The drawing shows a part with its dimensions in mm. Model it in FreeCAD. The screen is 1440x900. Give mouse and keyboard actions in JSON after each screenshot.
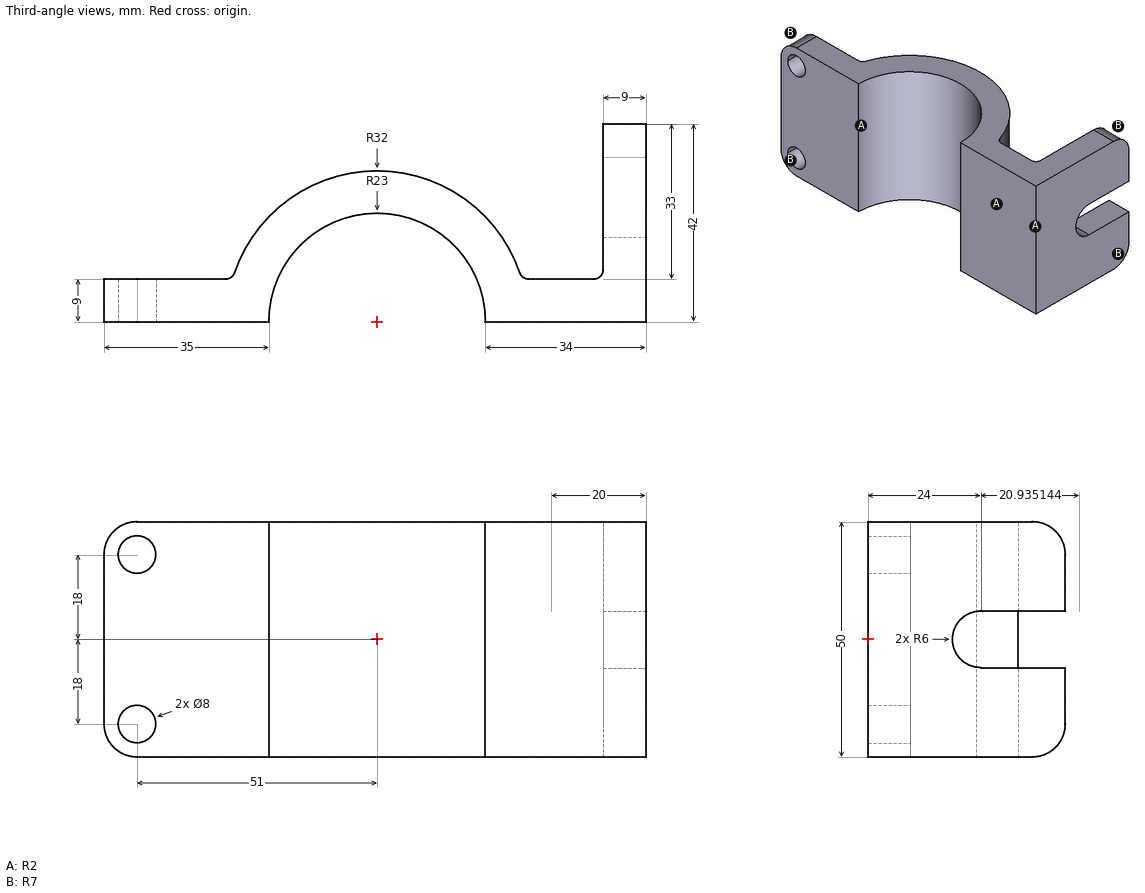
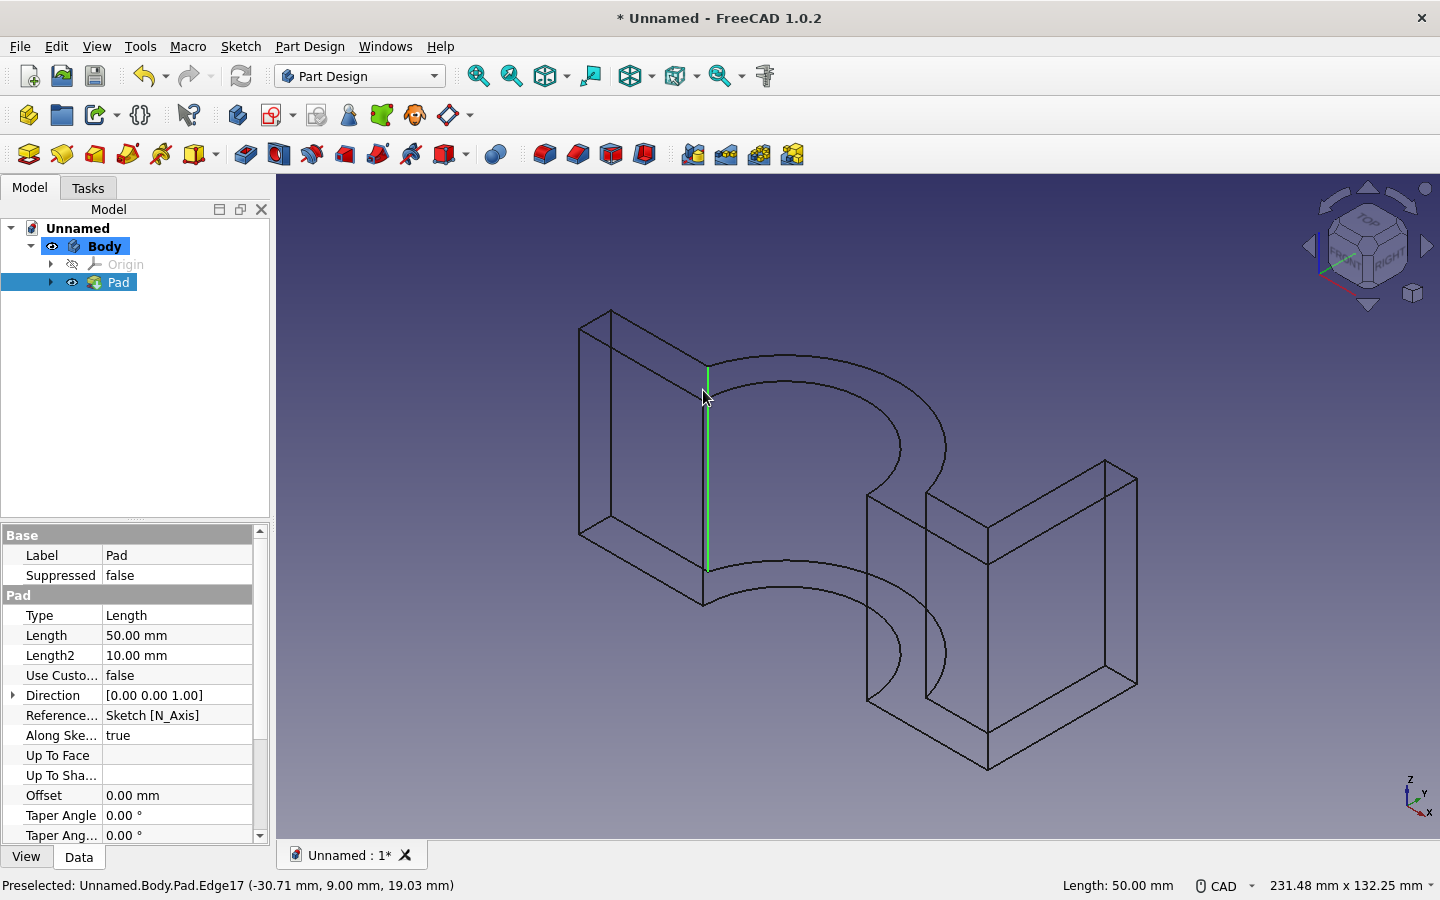
{"action": "left_click", "coordinate": [926, 594], "text": "ctrl"}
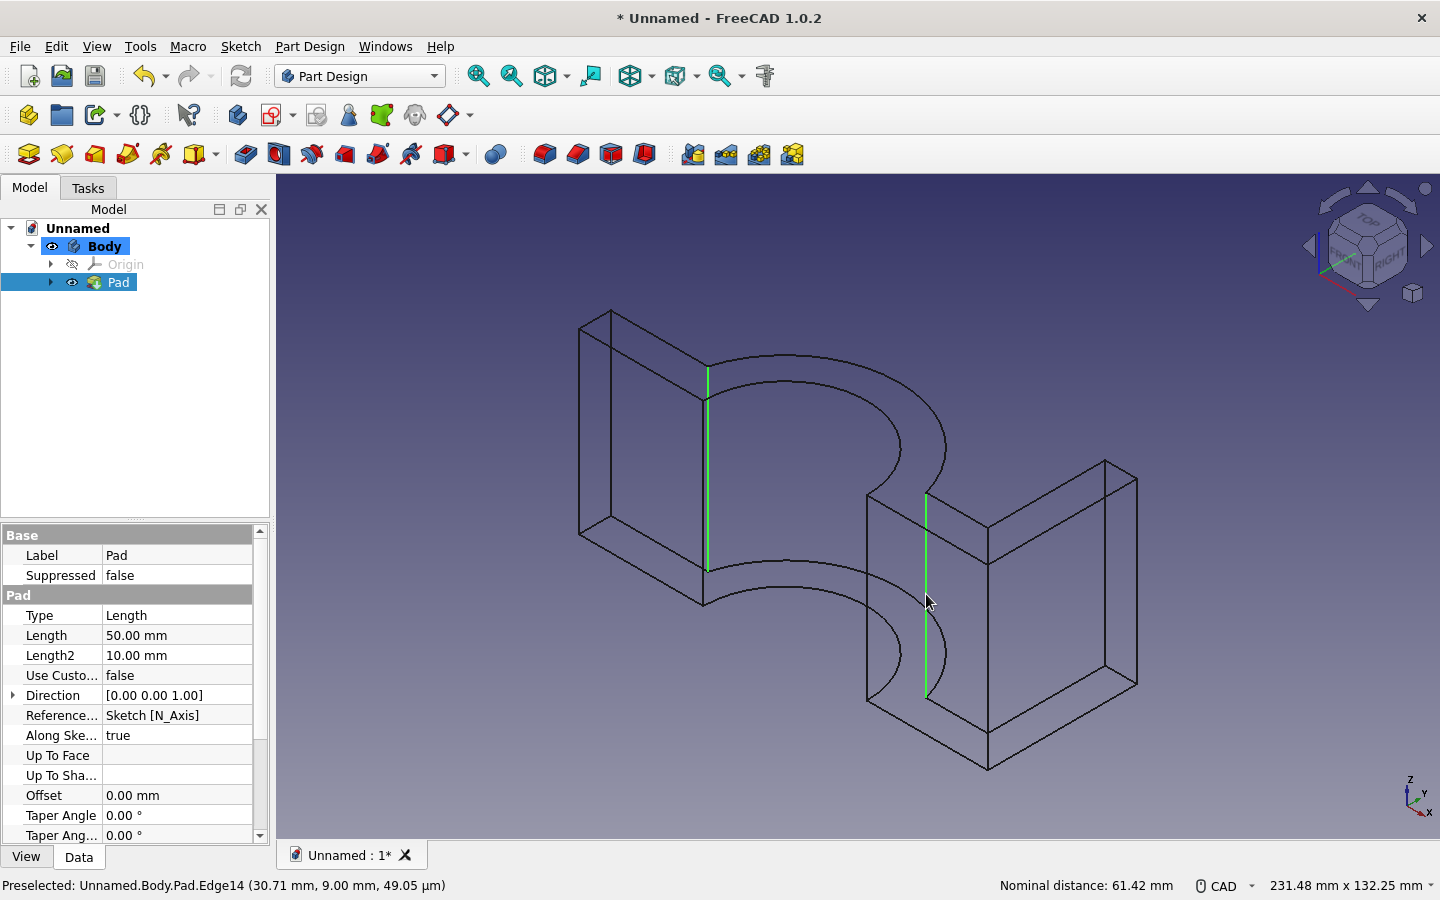
{"action": "left_click", "coordinate": [988, 552], "text": "ctrl"}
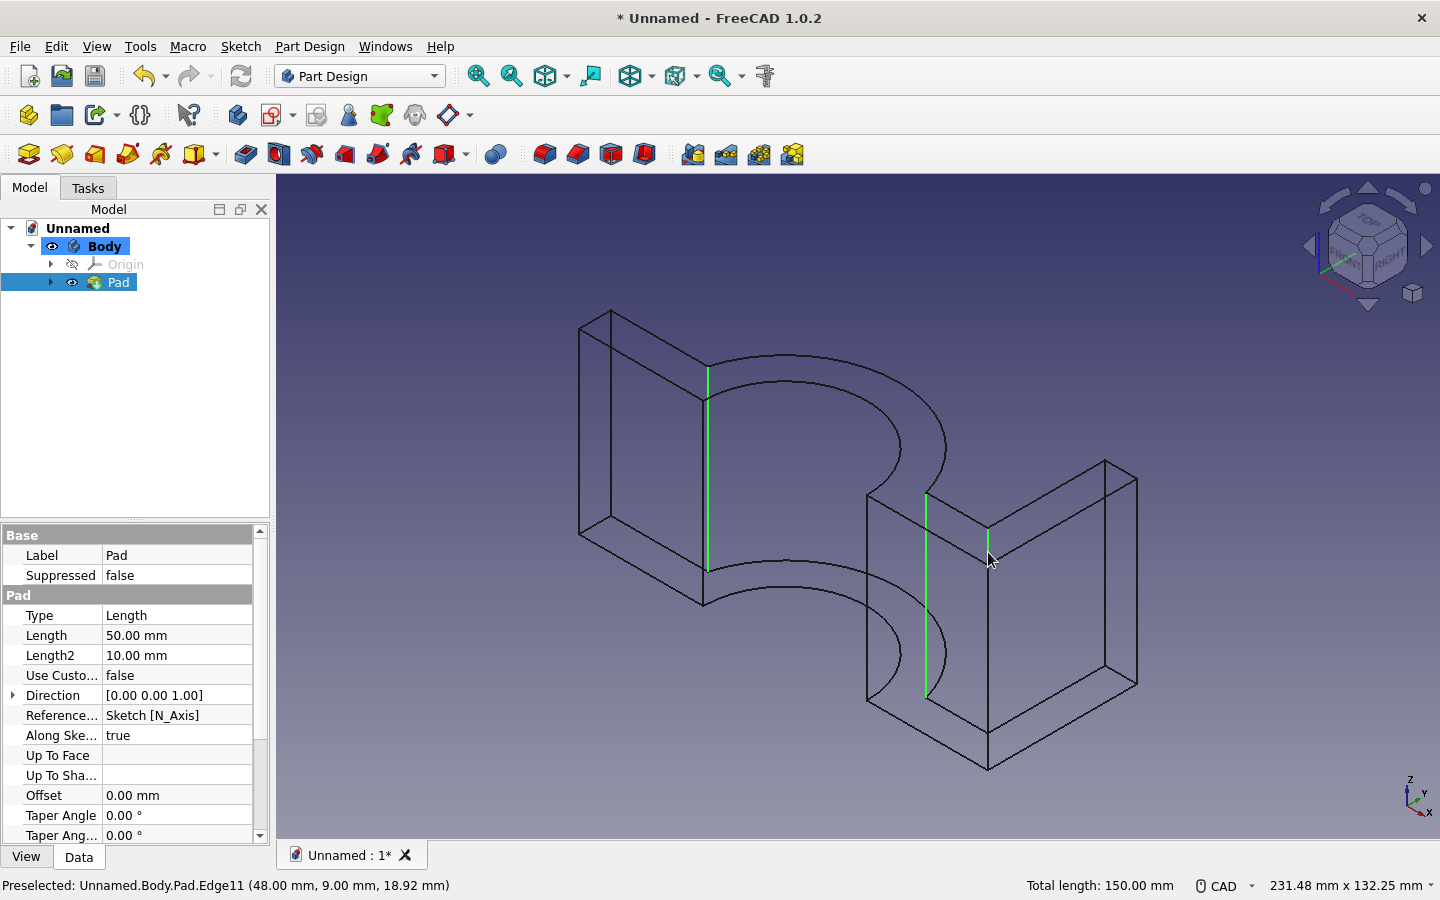
{"action": "key", "text": "v 1"}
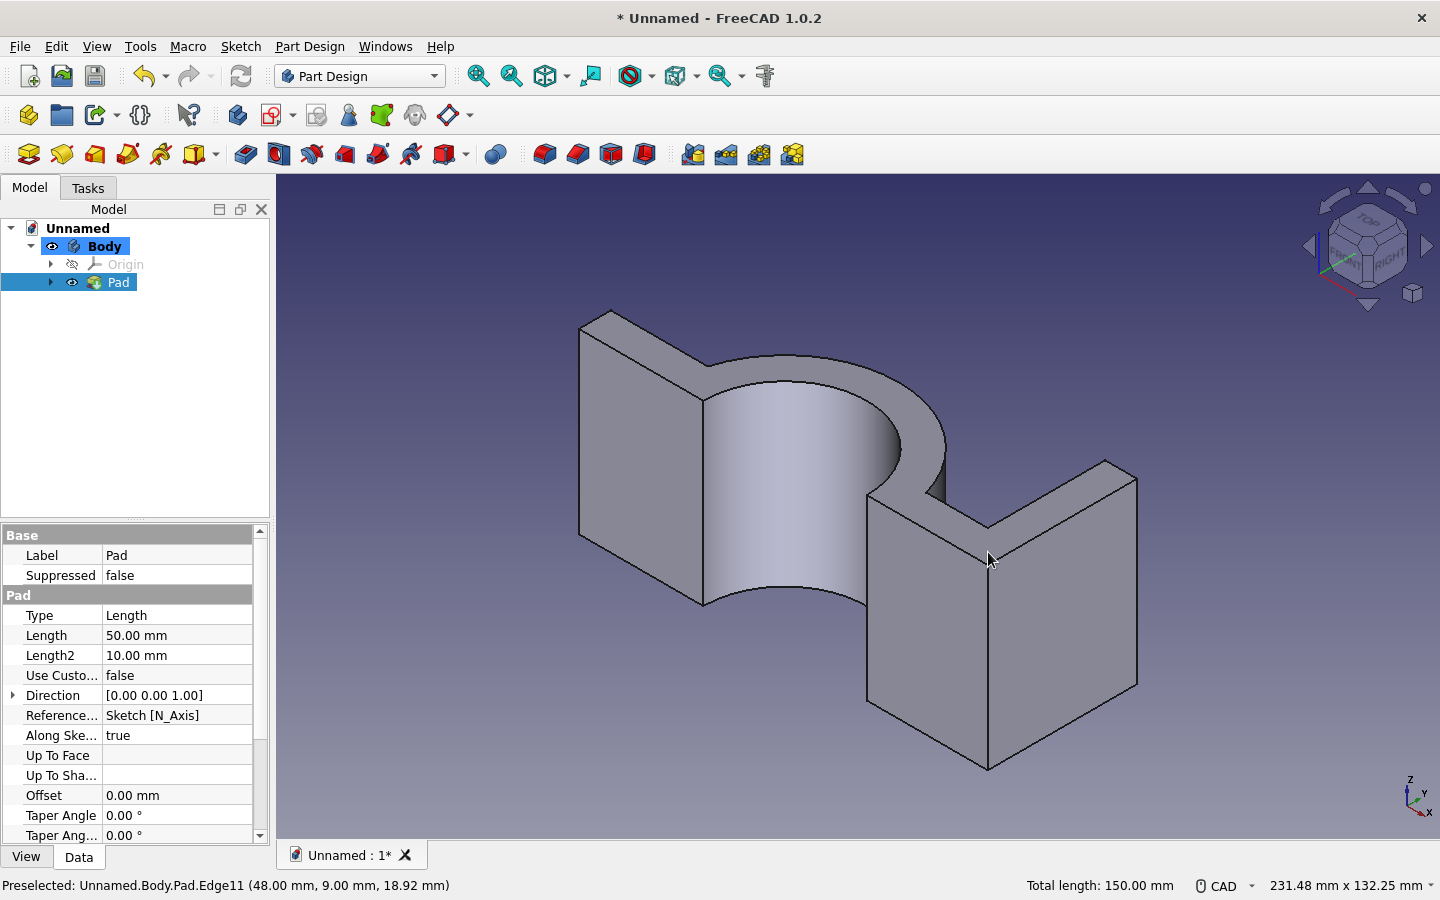
{"action": "left_click", "coordinate": [545, 154]}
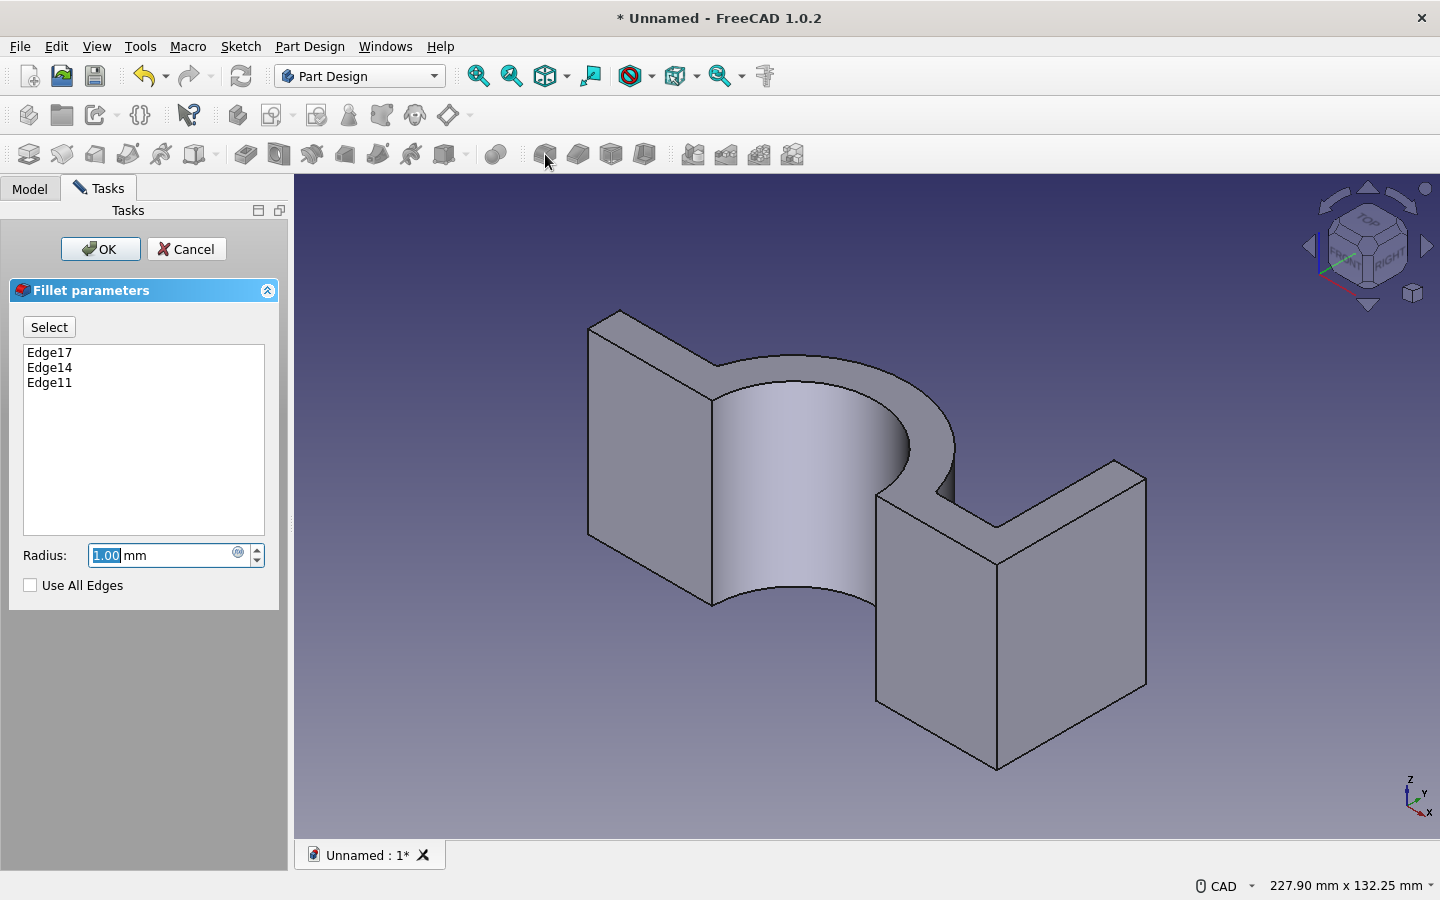
{"action": "type", "text": "2"}
{"action": "key", "text": "Tab"}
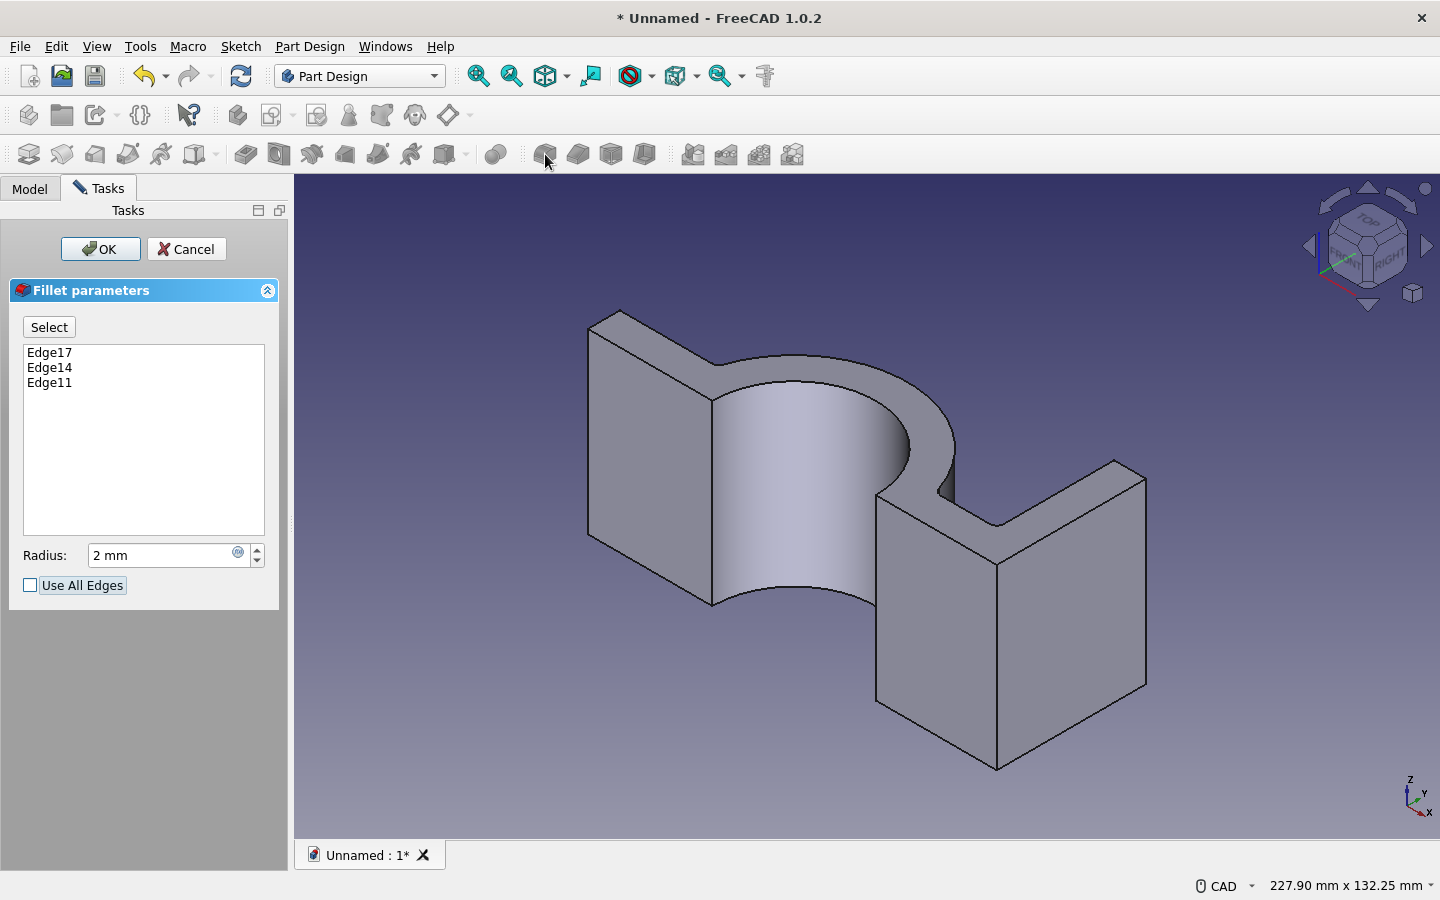
{"action": "left_click", "coordinate": [101, 249]}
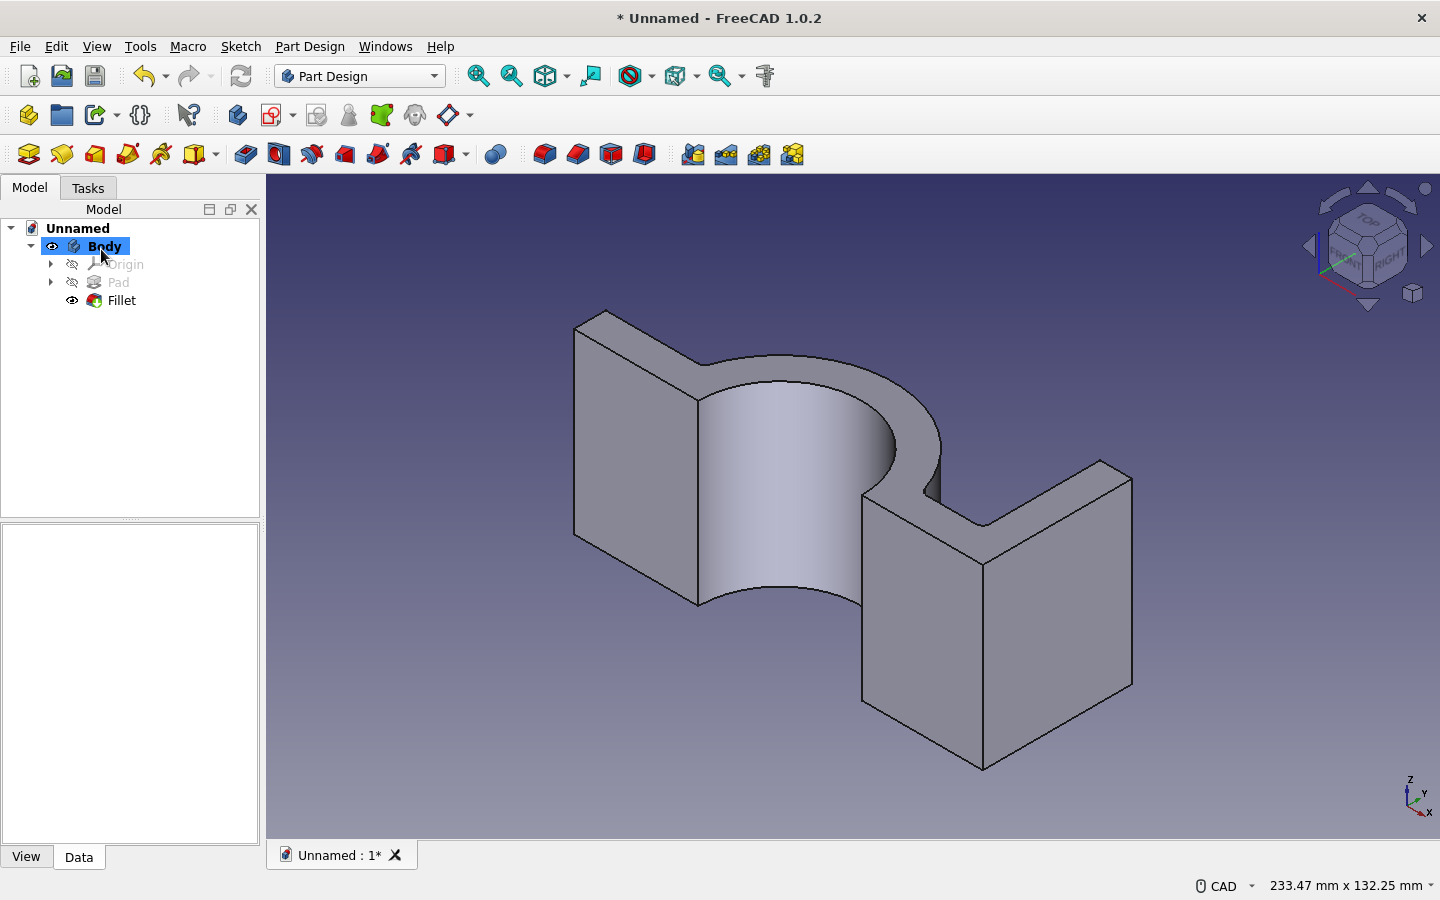
{"action": "key", "text": "2"}